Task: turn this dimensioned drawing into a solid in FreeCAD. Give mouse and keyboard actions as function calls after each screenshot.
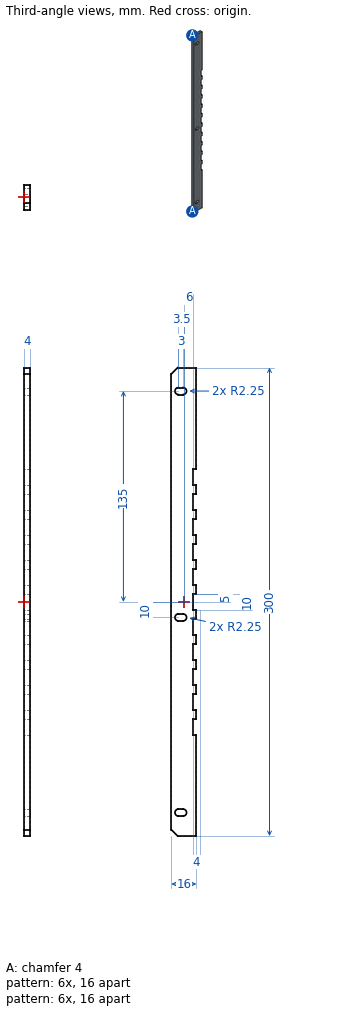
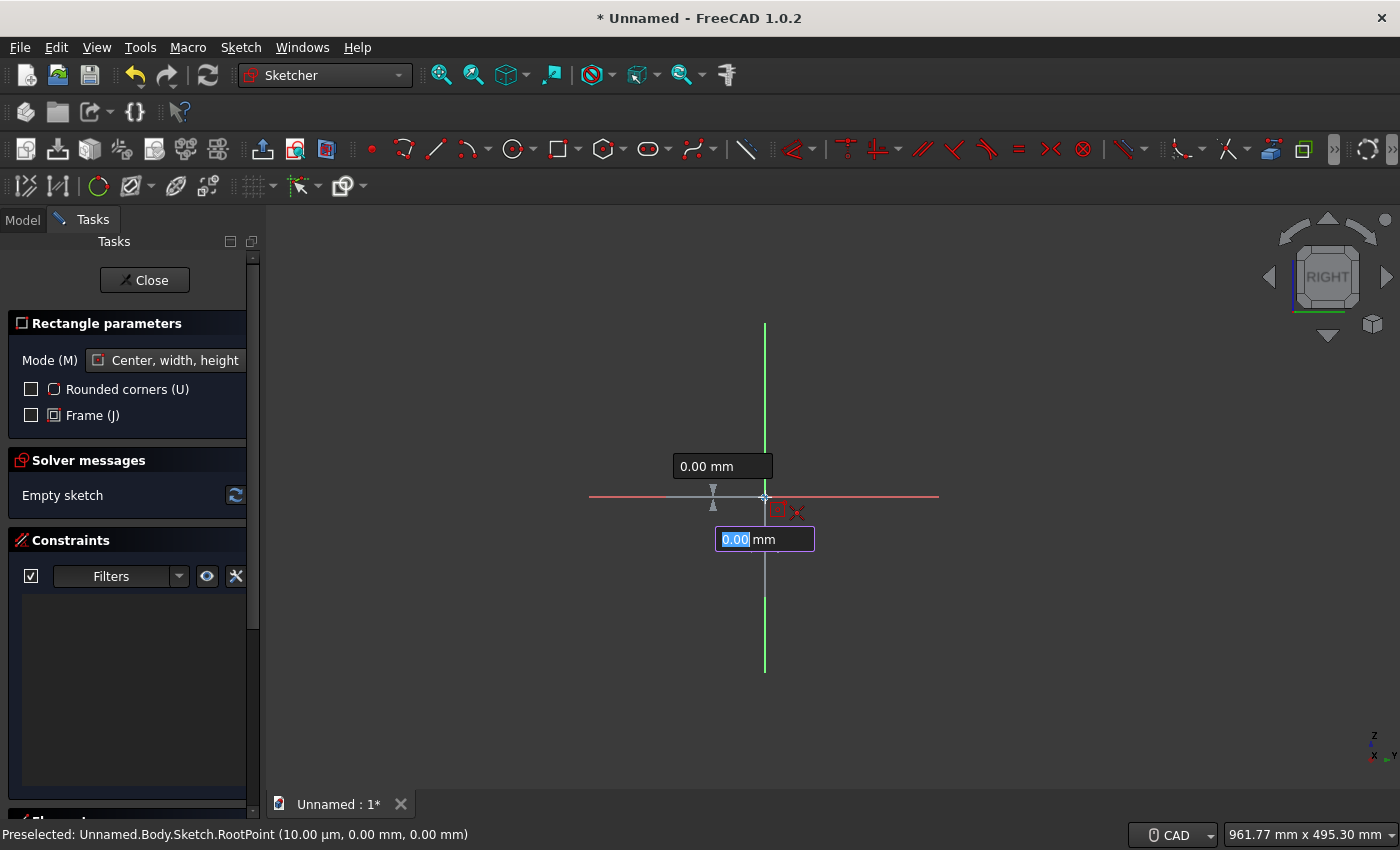
scroll(774, 321, up, 3)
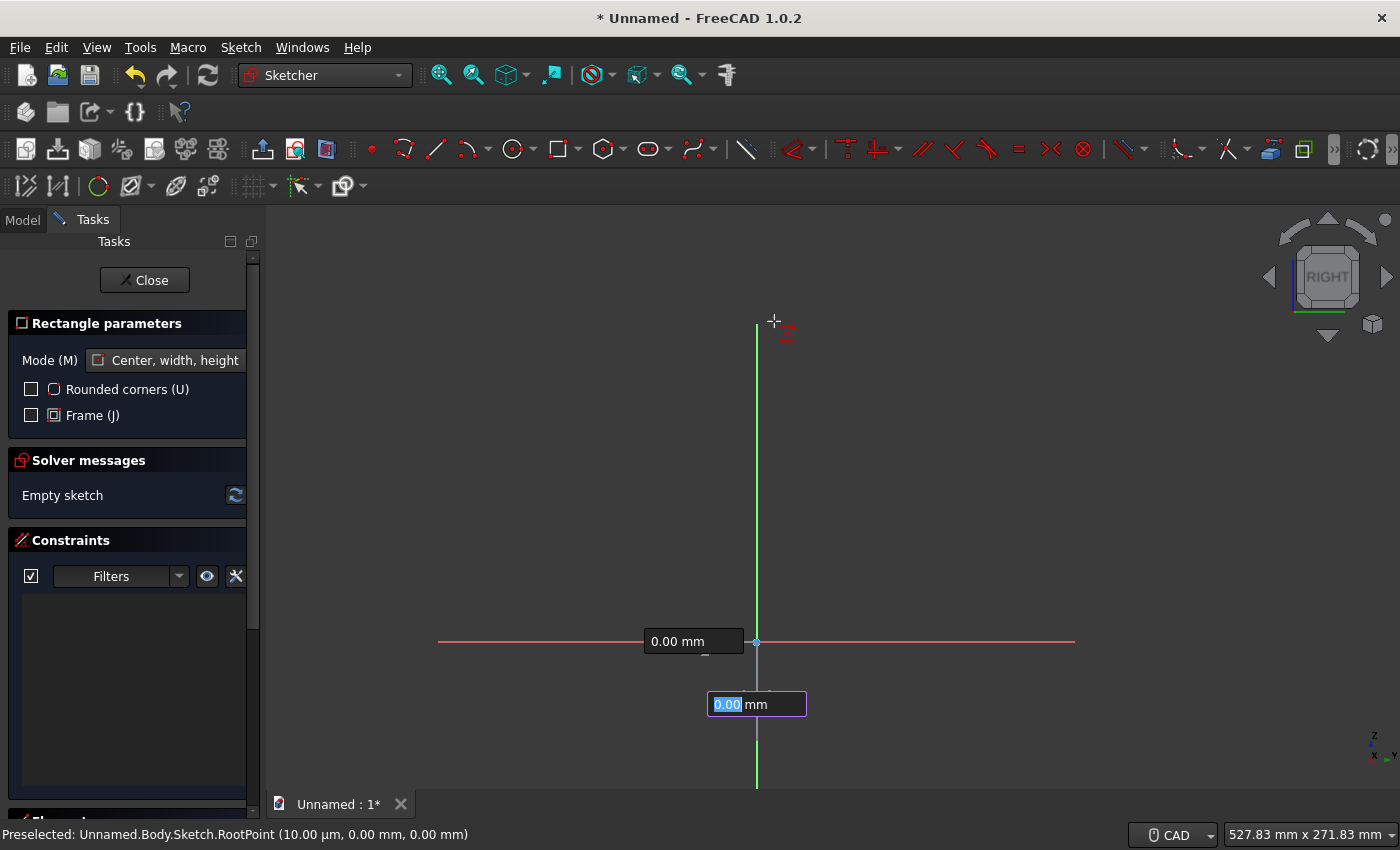
click(774, 320)
key(Escape)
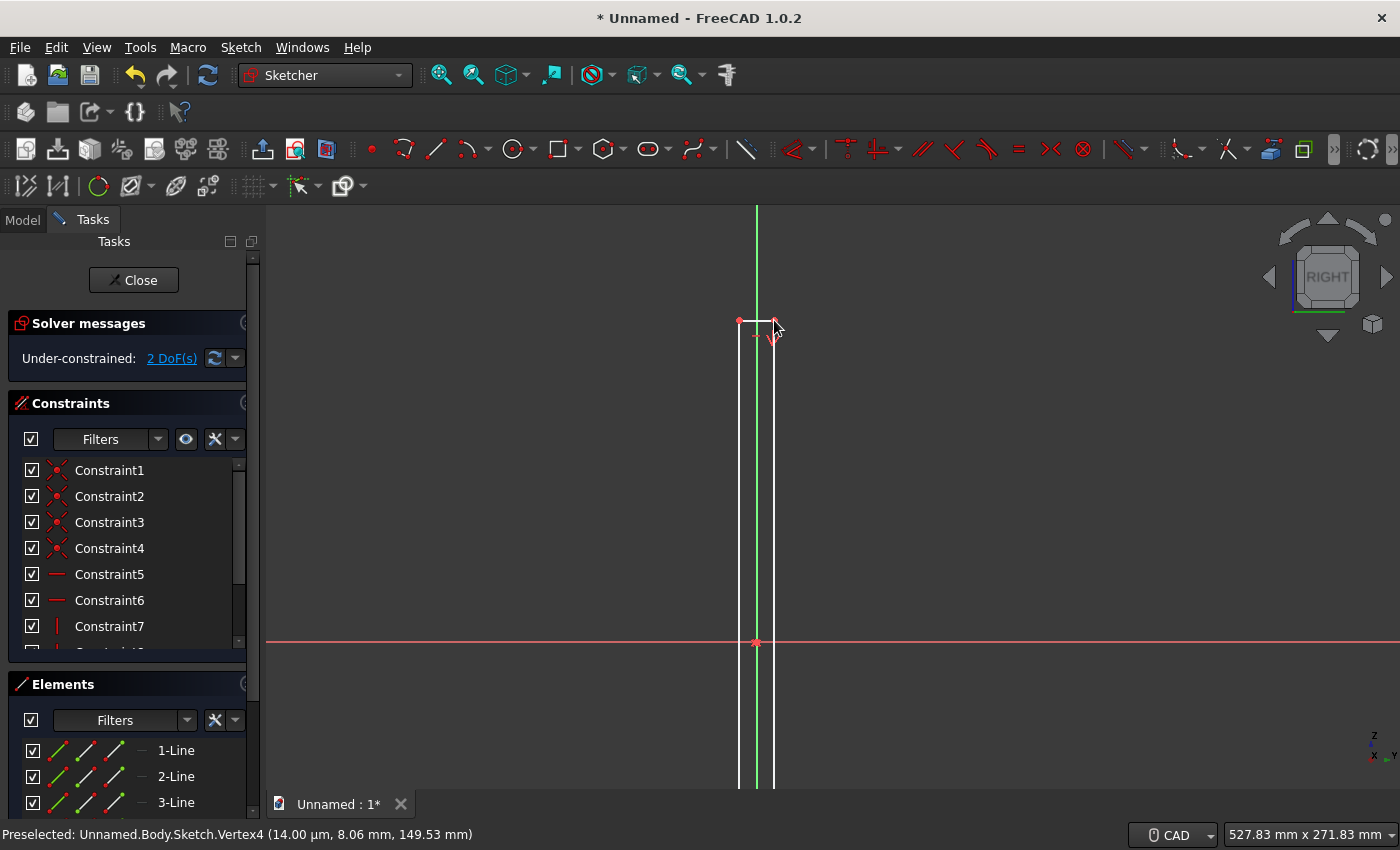
scroll(774, 320, down, 3)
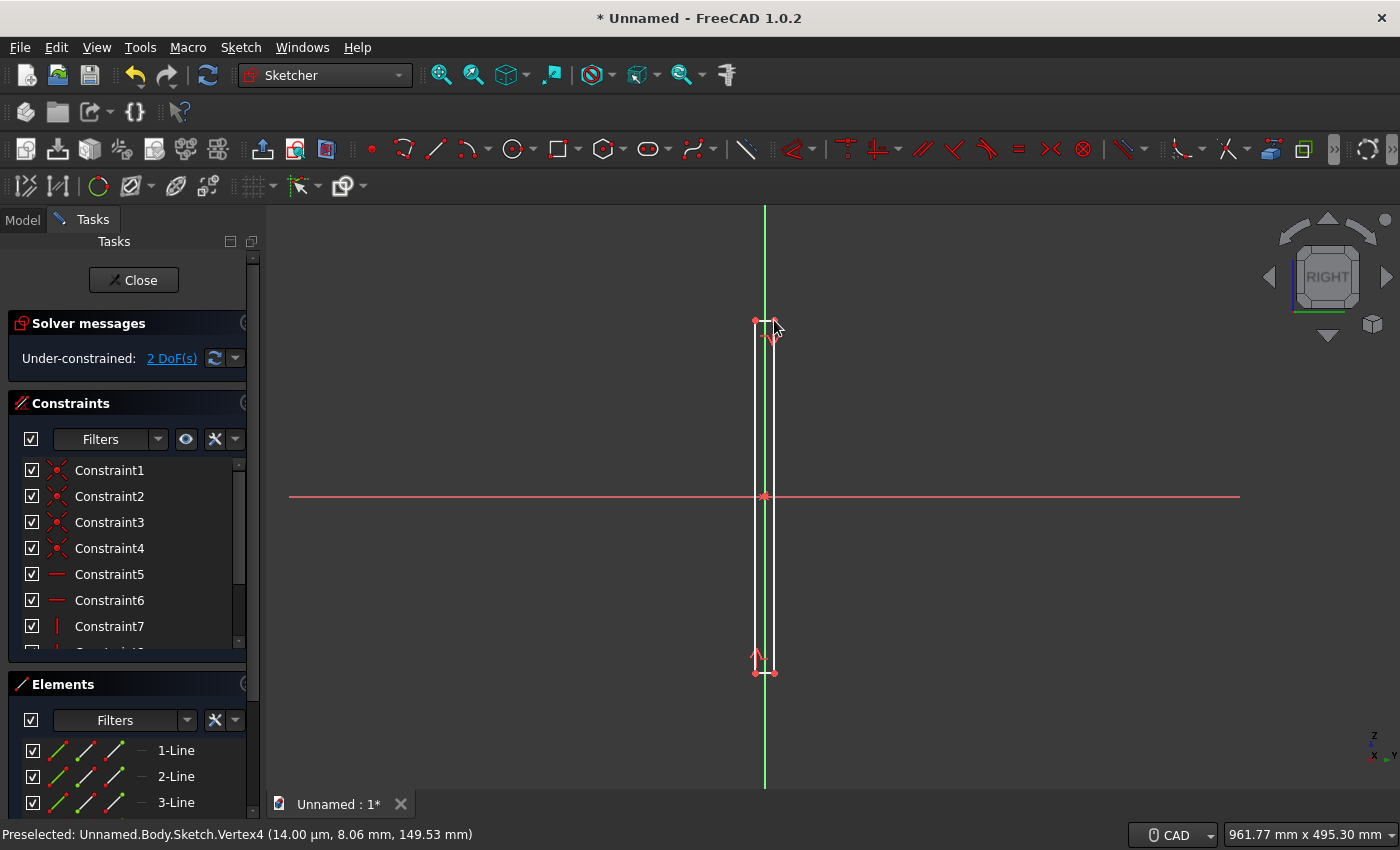
scroll(763, 673, up, 4)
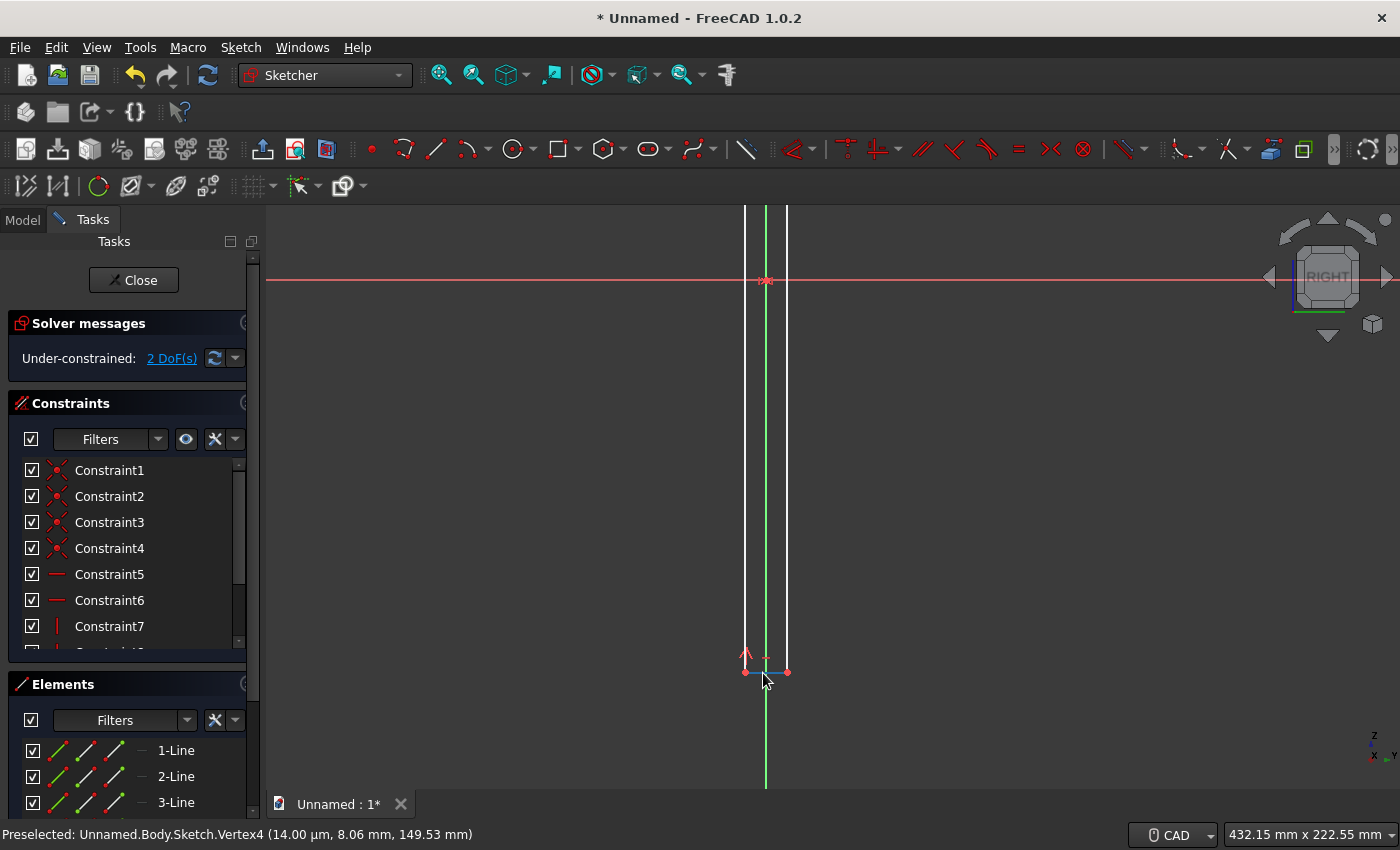
click(762, 673)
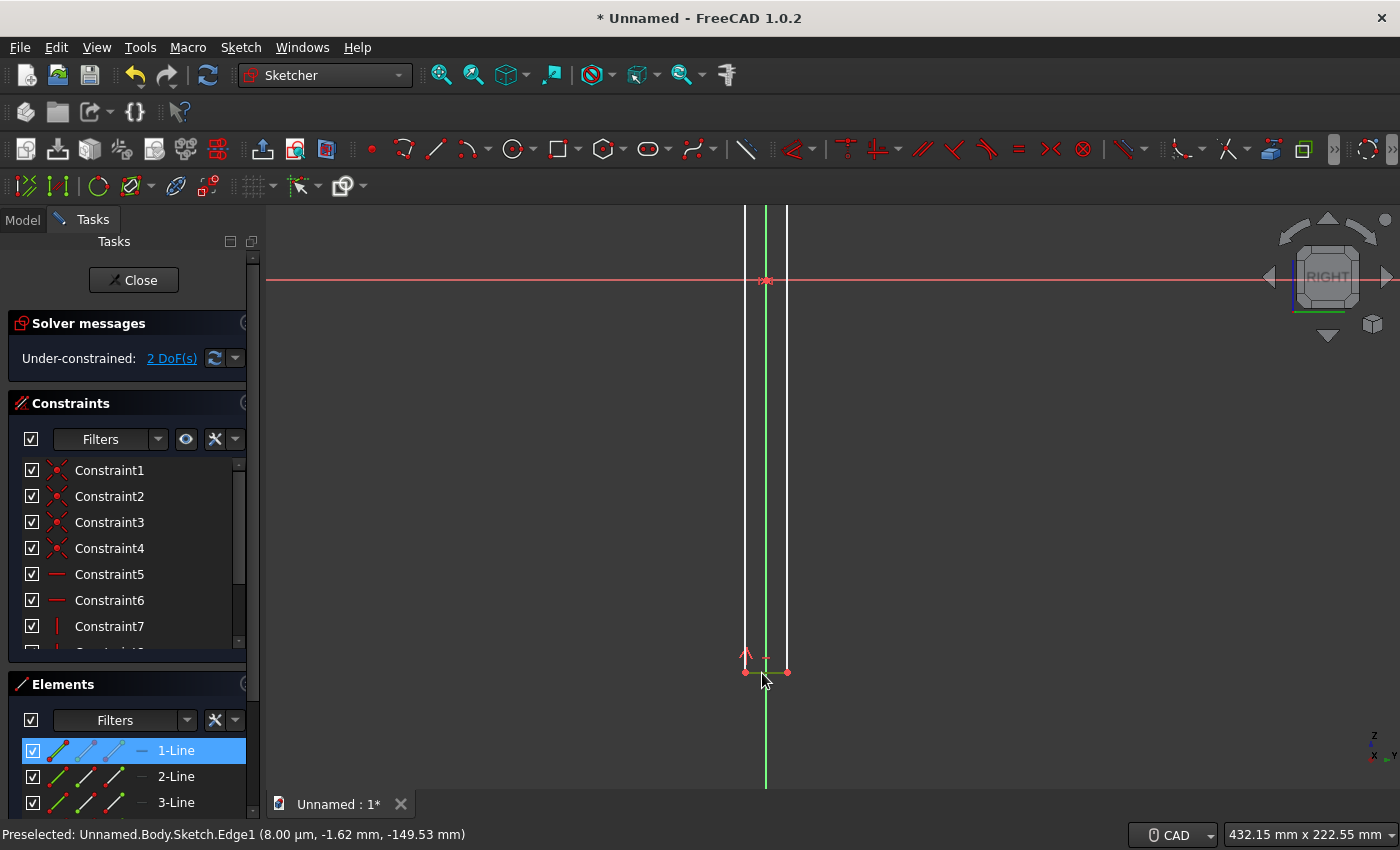
click(814, 150)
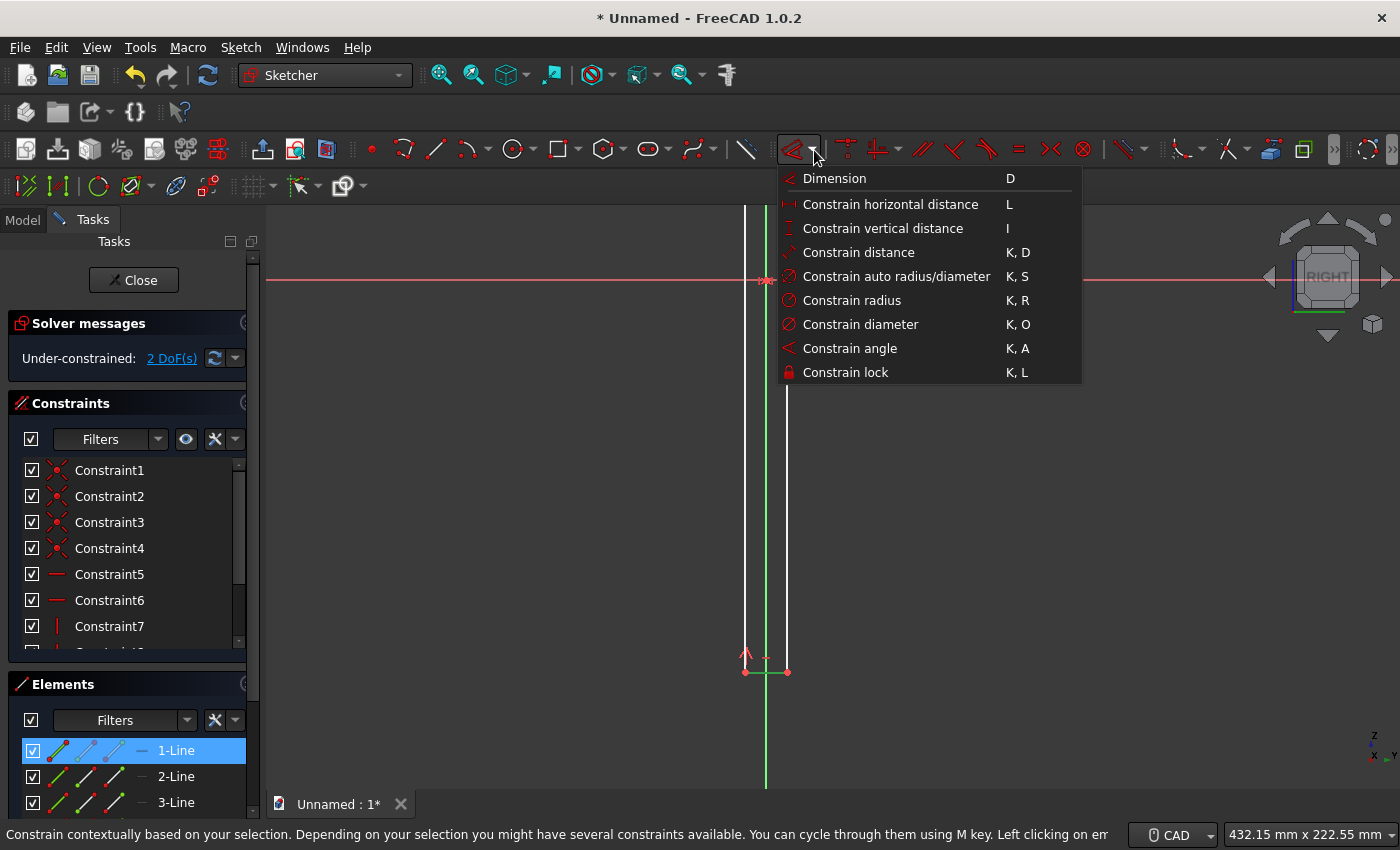
click(930, 204)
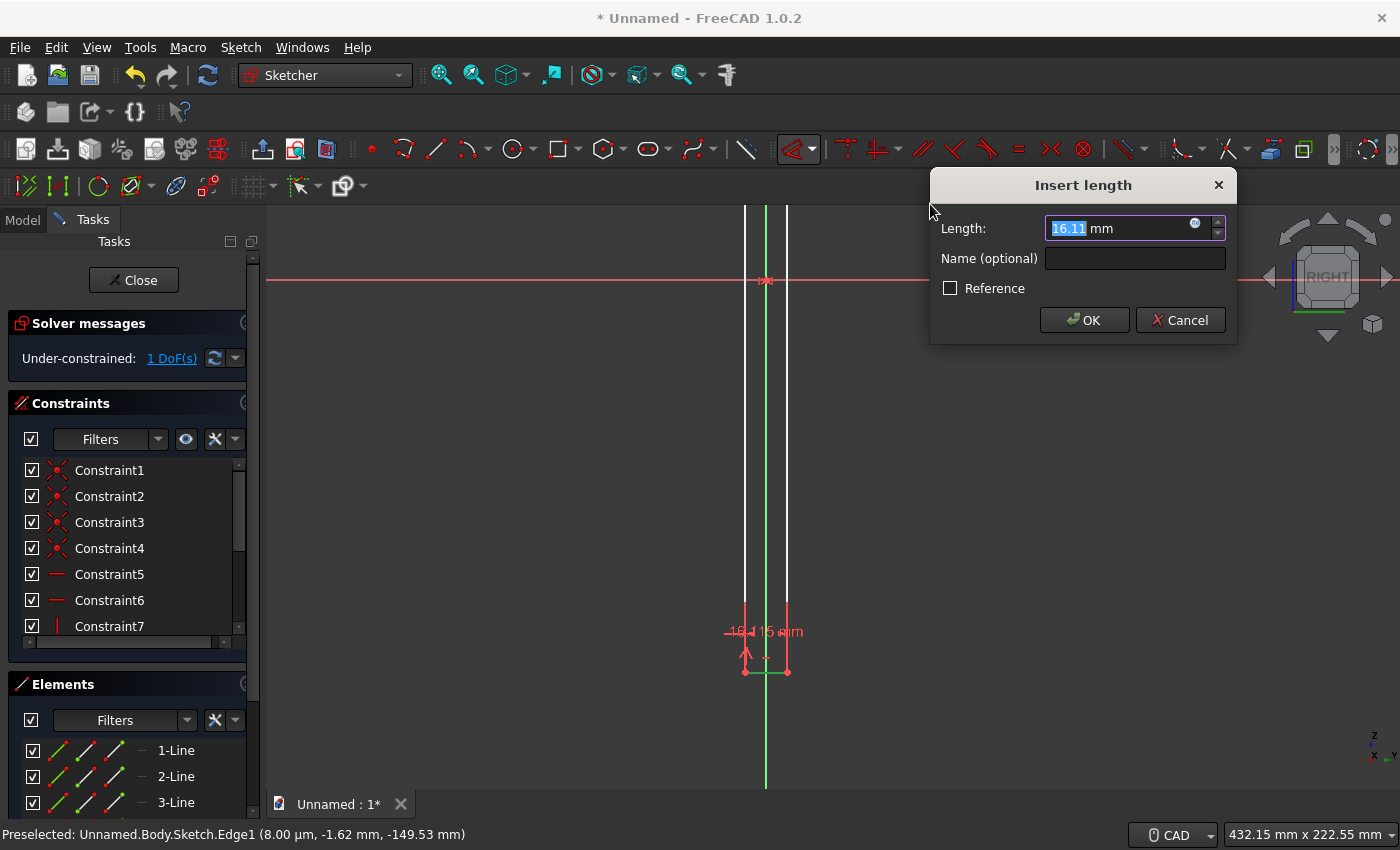
text(16)
key(Return)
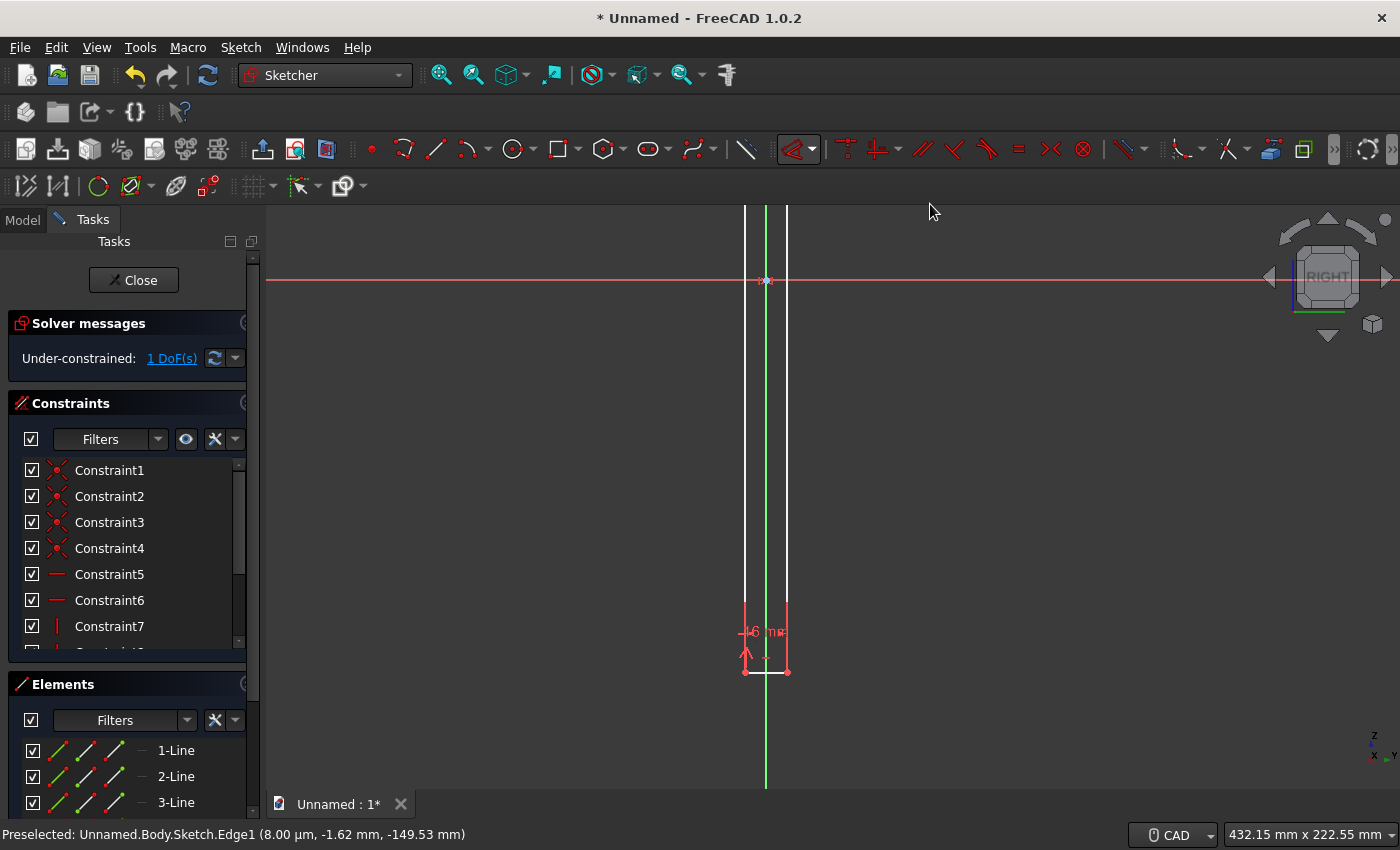
click(787, 437)